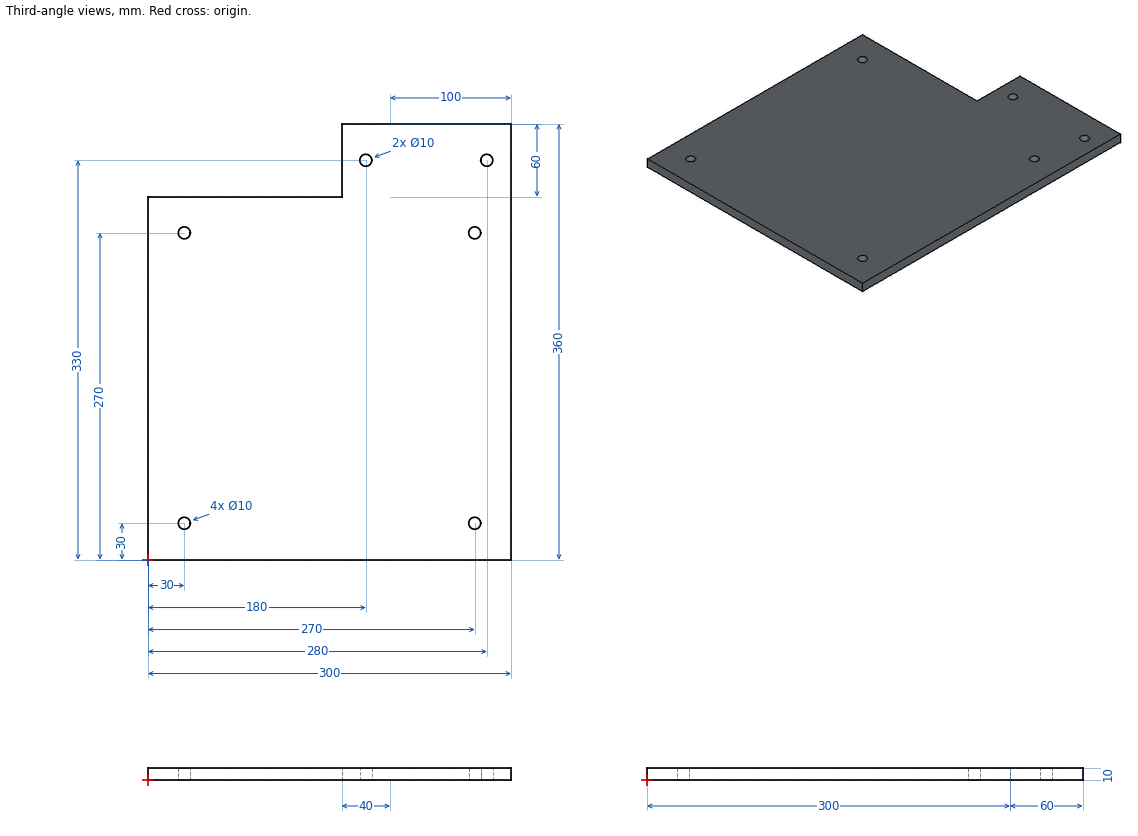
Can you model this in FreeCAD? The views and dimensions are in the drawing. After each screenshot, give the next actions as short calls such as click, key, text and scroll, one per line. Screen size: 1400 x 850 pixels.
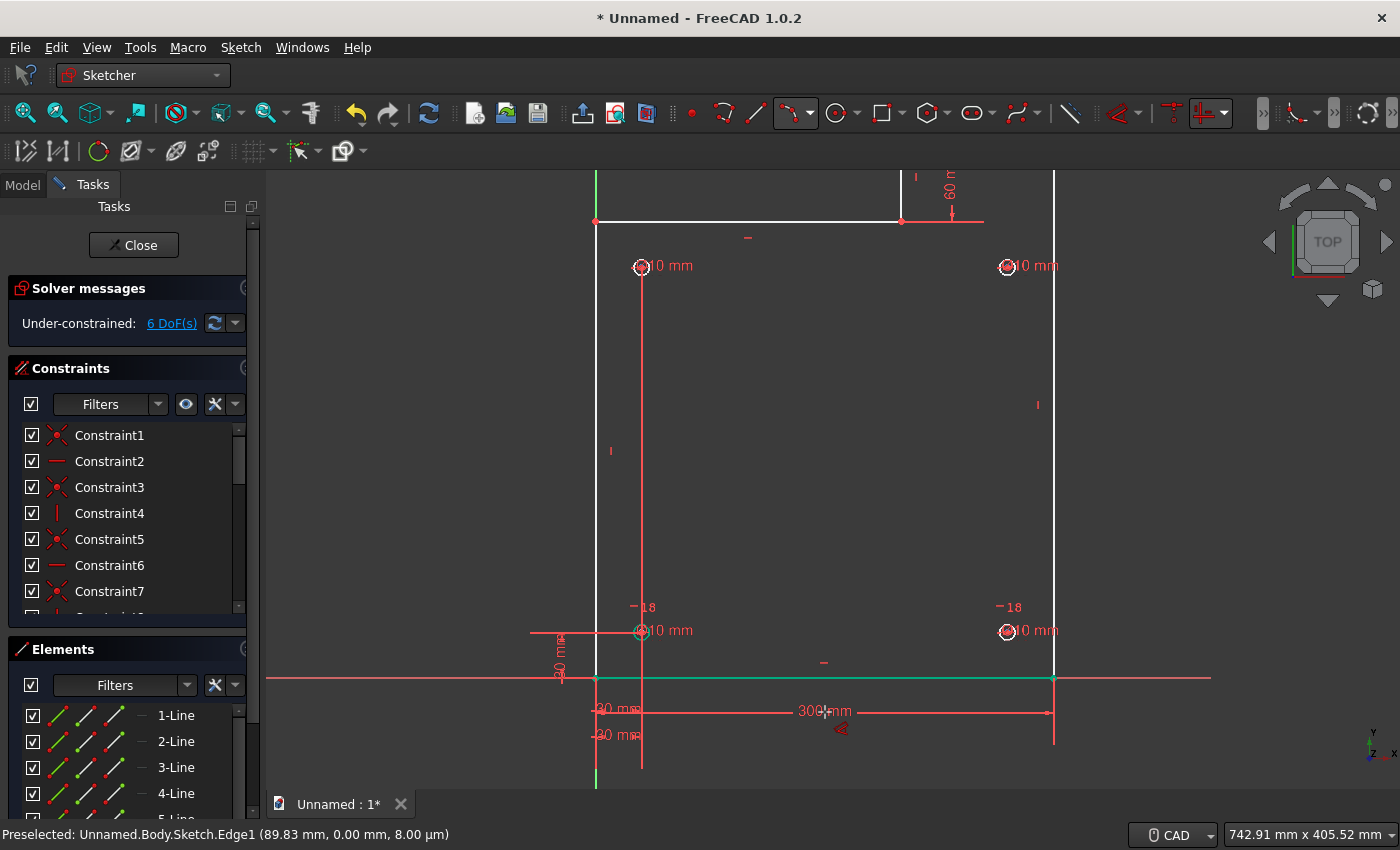
click(1054, 514)
click(1088, 438)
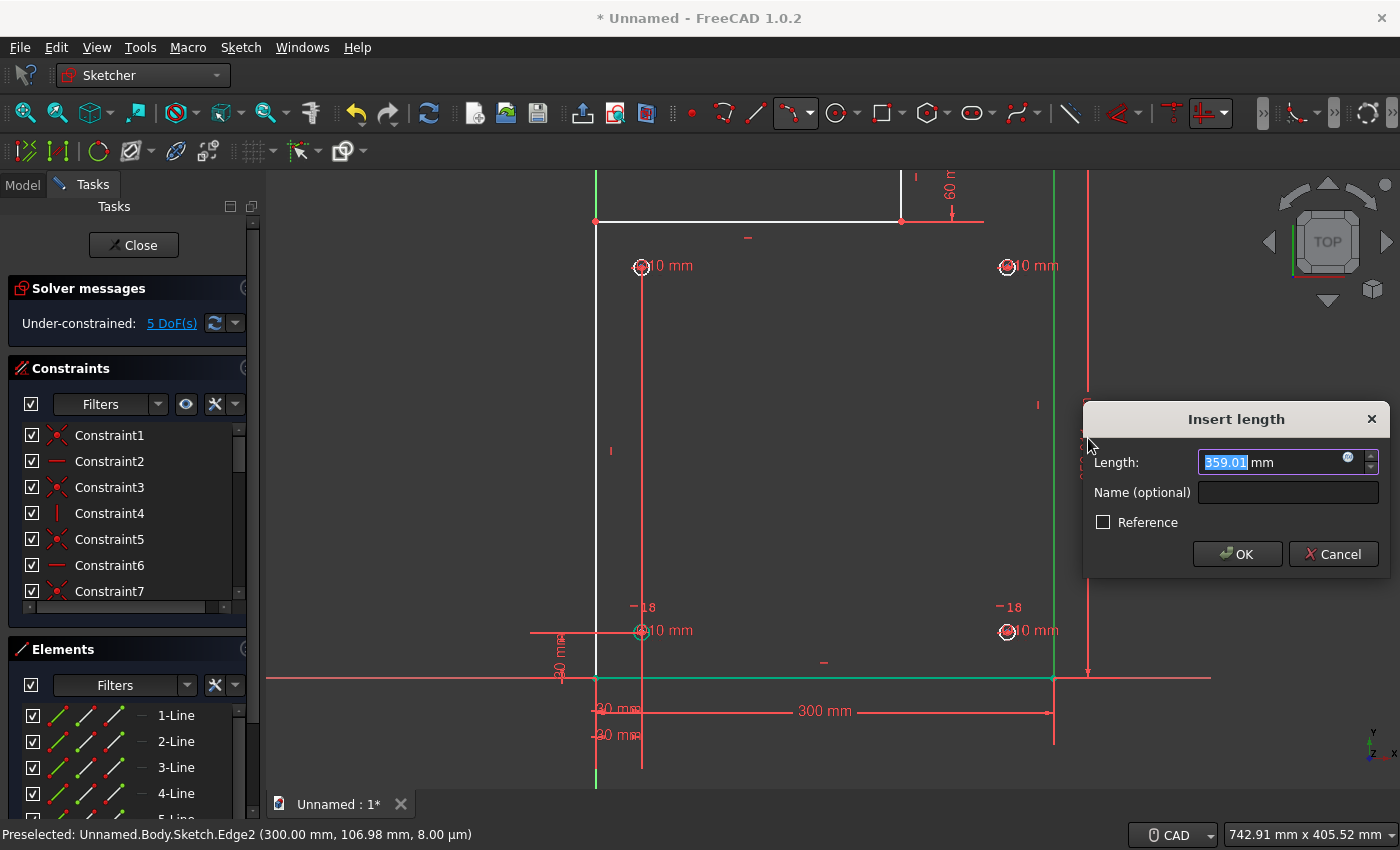
text(360)
key(Return)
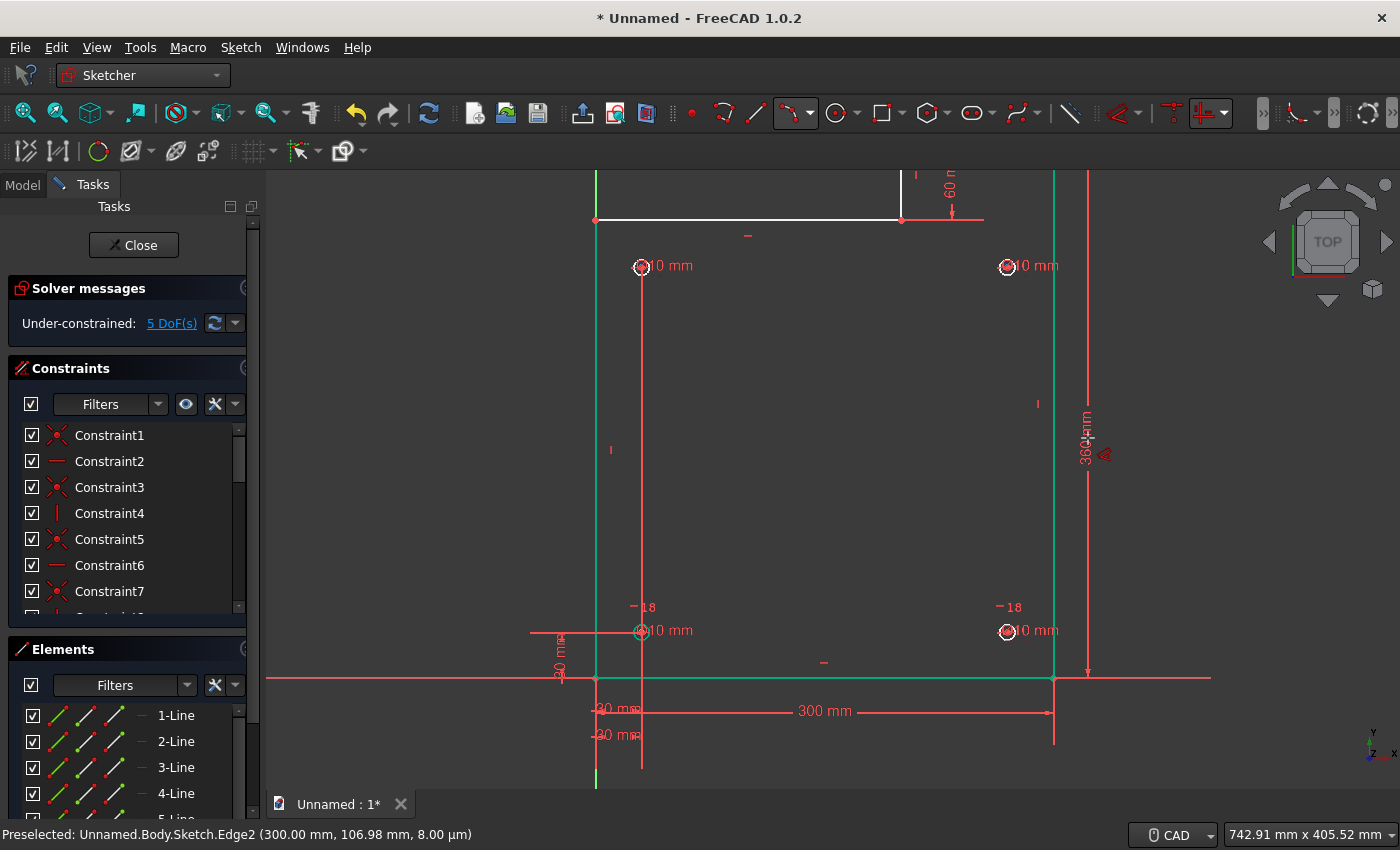
scroll(642, 634, down, 2)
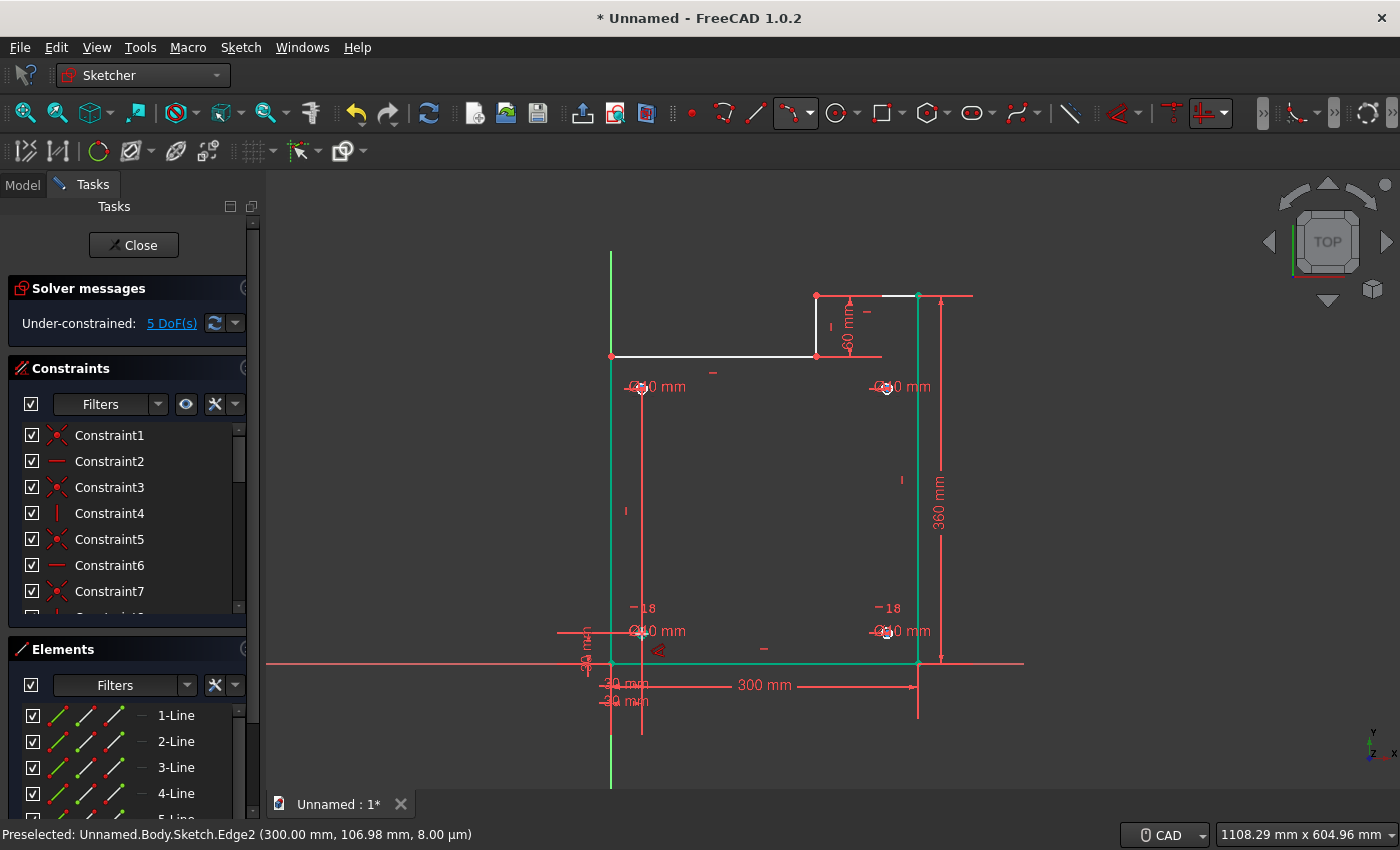
click(888, 296)
click(867, 262)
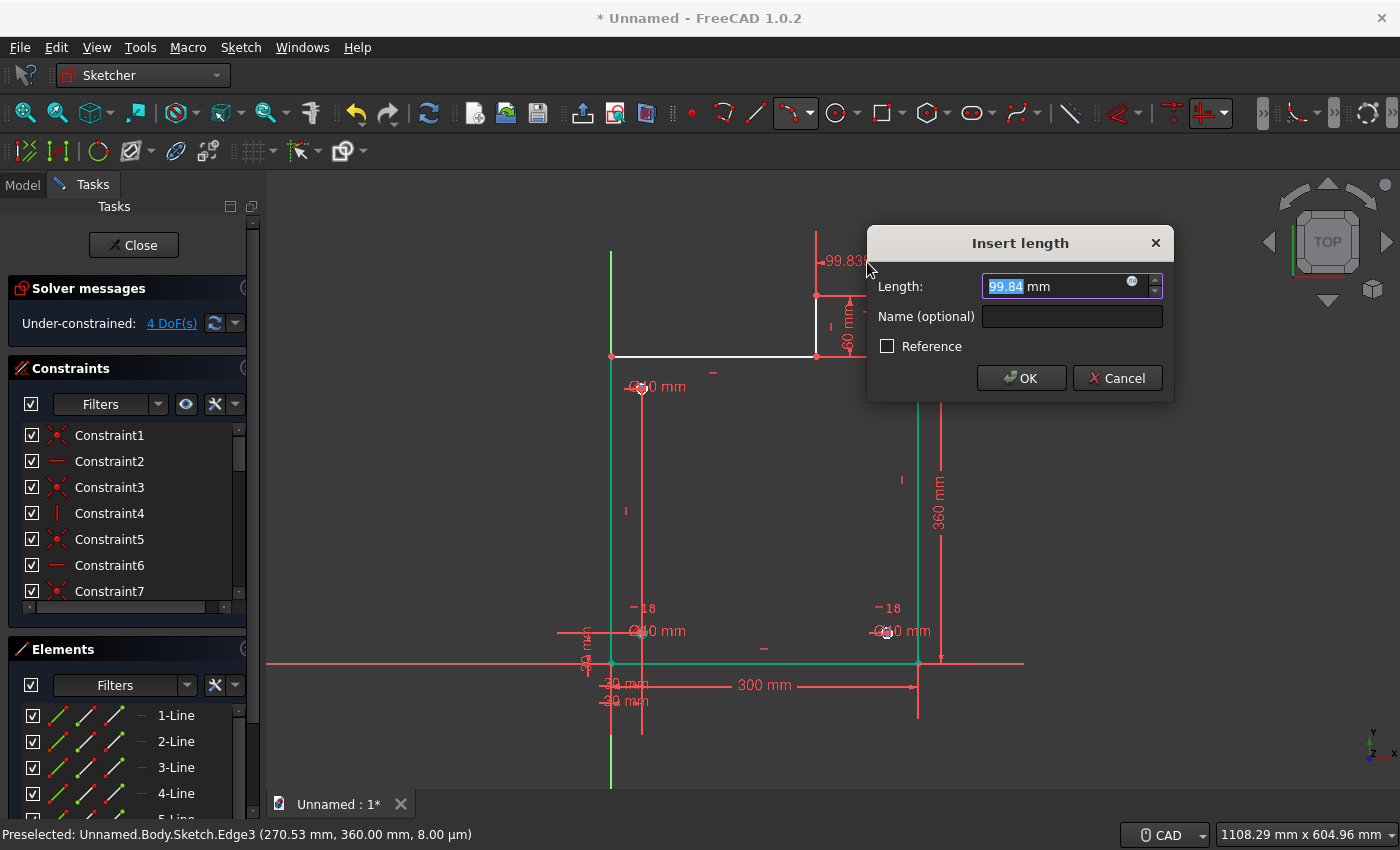
text(100)
key(Return)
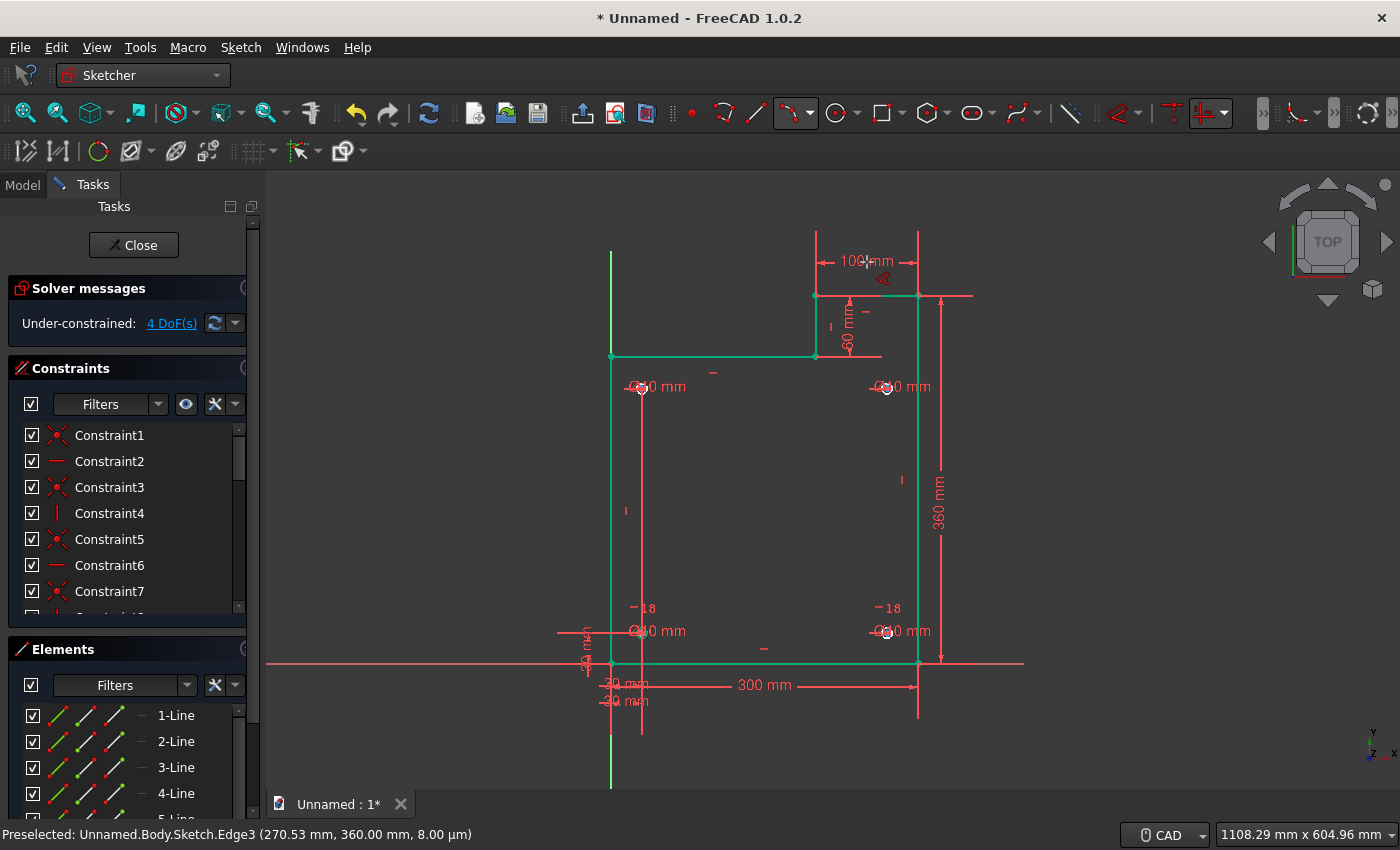
click(887, 633)
click(846, 698)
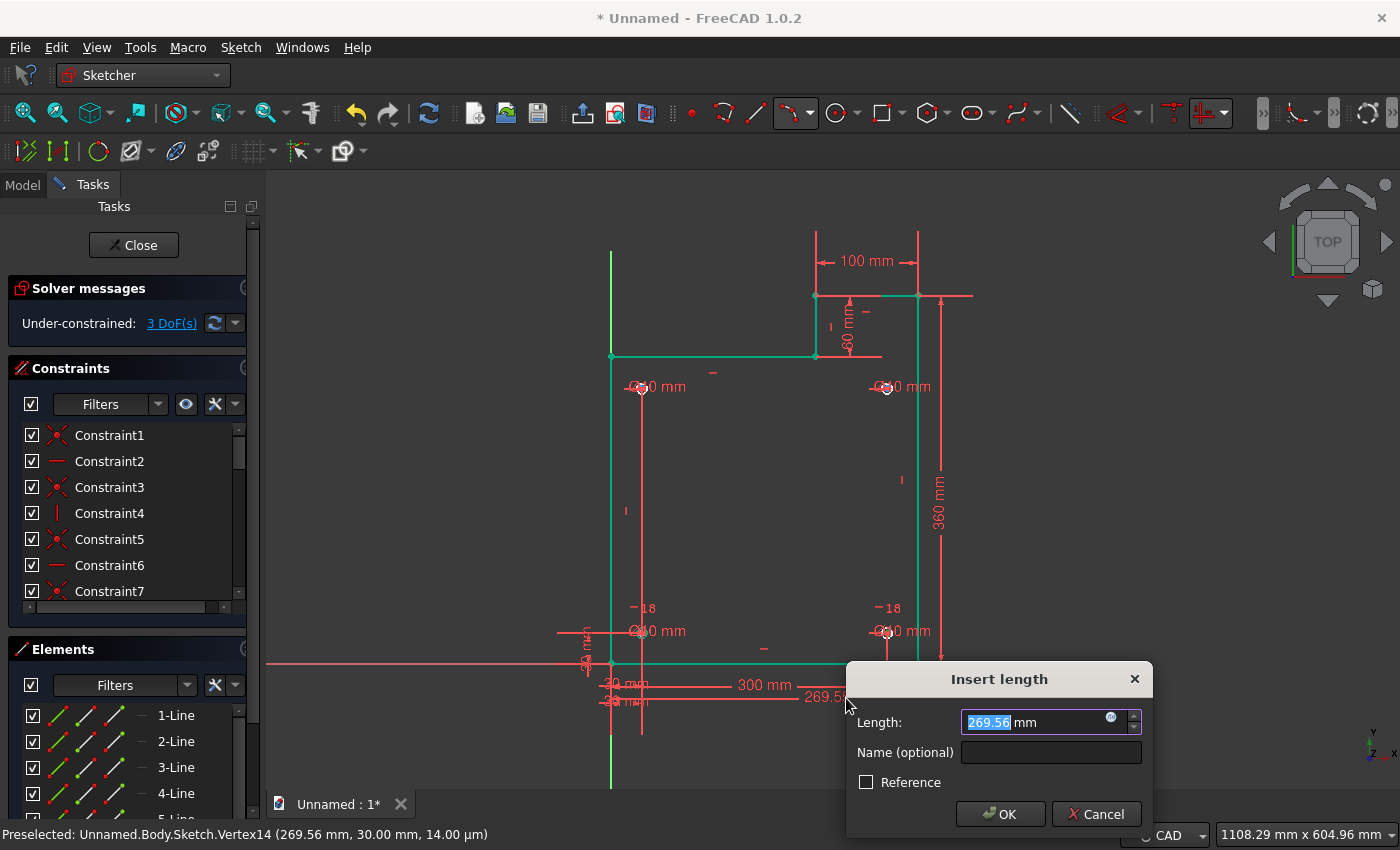
text(270)
key(Return)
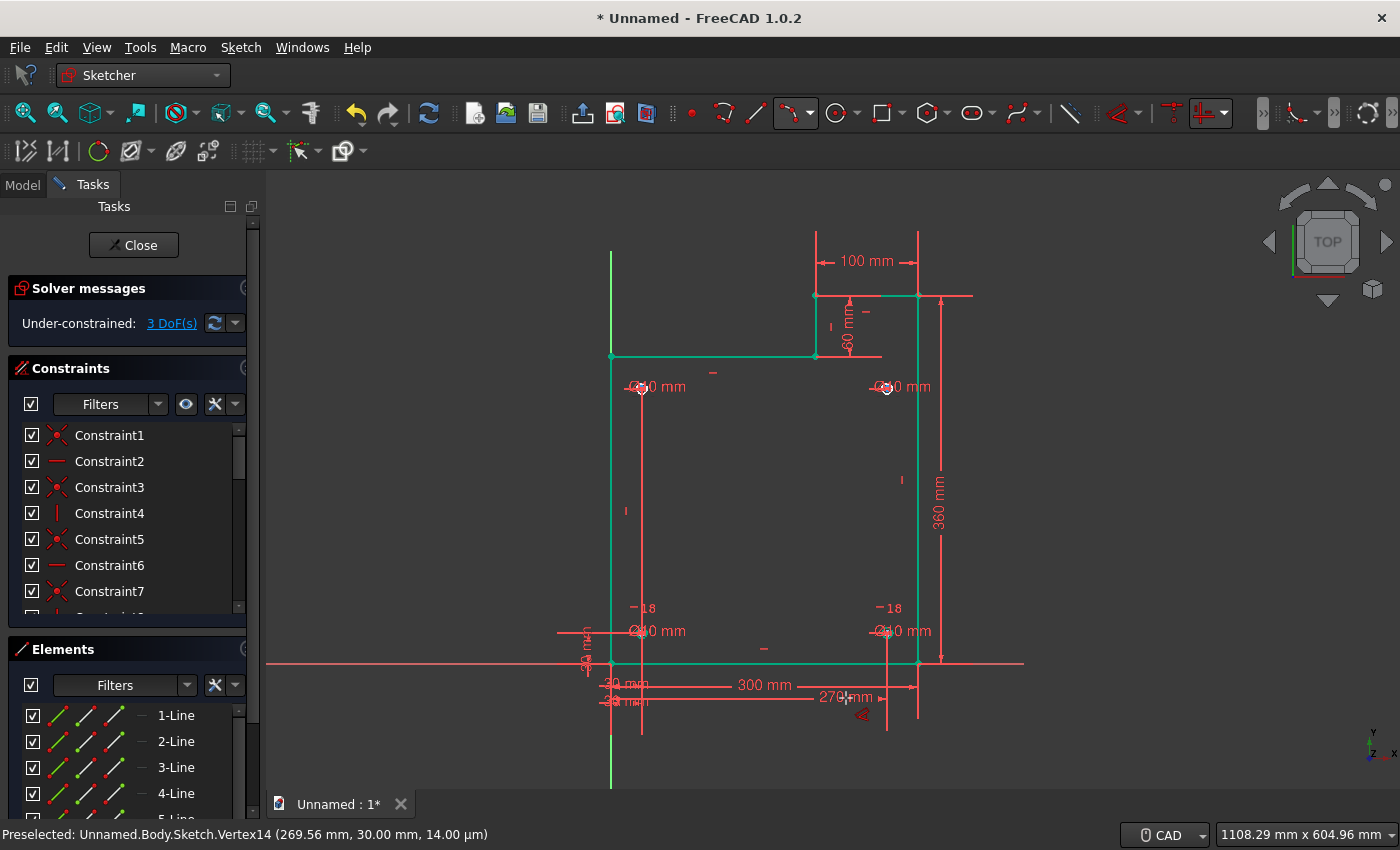
click(642, 389)
click(577, 526)